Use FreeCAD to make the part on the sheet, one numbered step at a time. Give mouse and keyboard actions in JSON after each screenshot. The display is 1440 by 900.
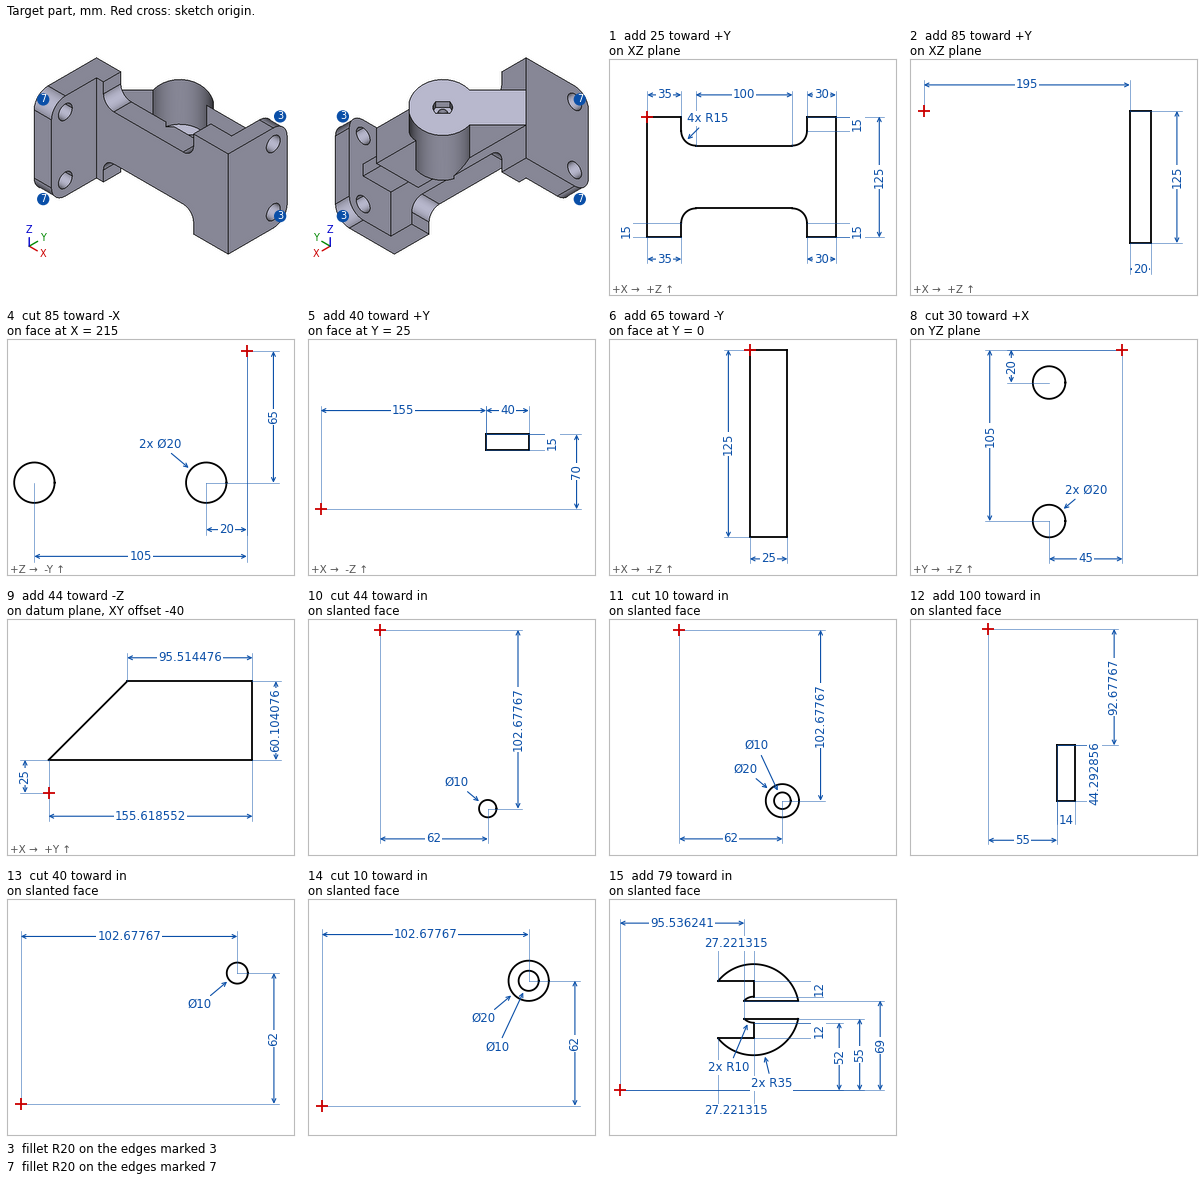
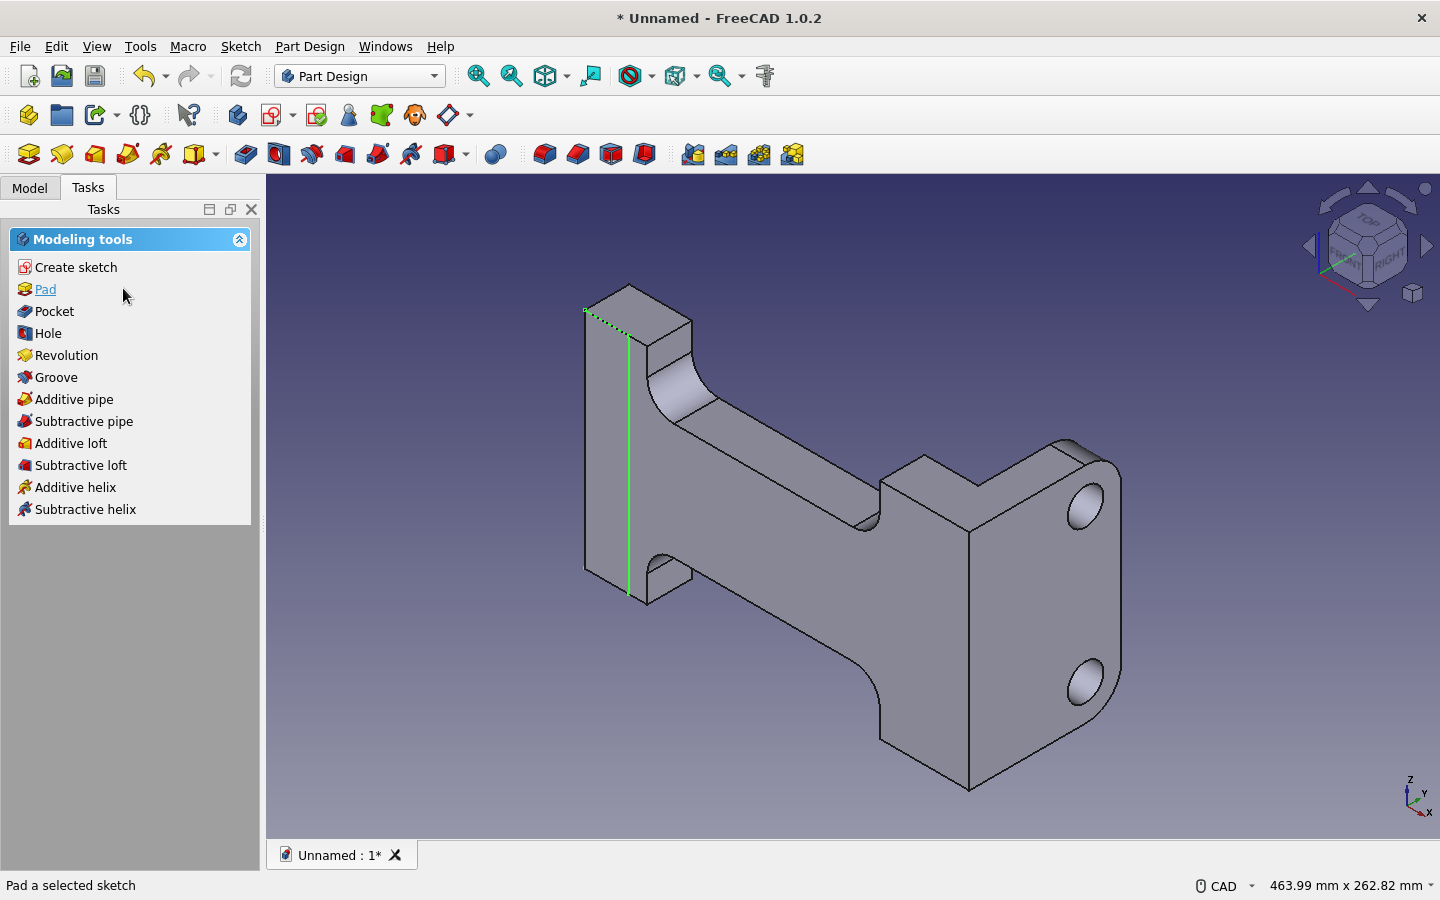
{"action": "left_click", "coordinate": [29, 154]}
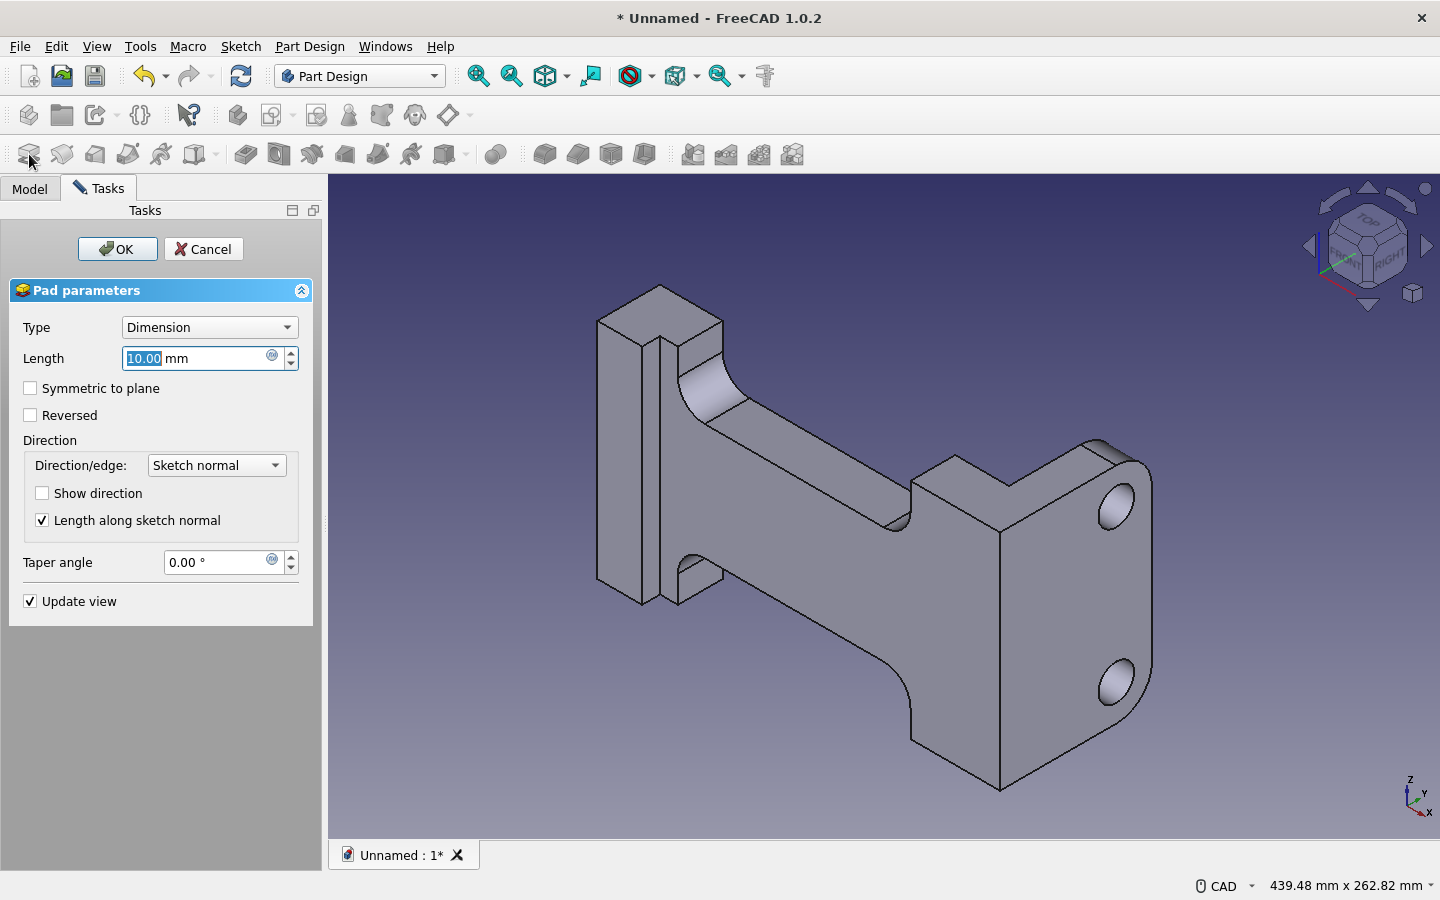
{"action": "type", "text": "65"}
{"action": "key", "text": "Tab"}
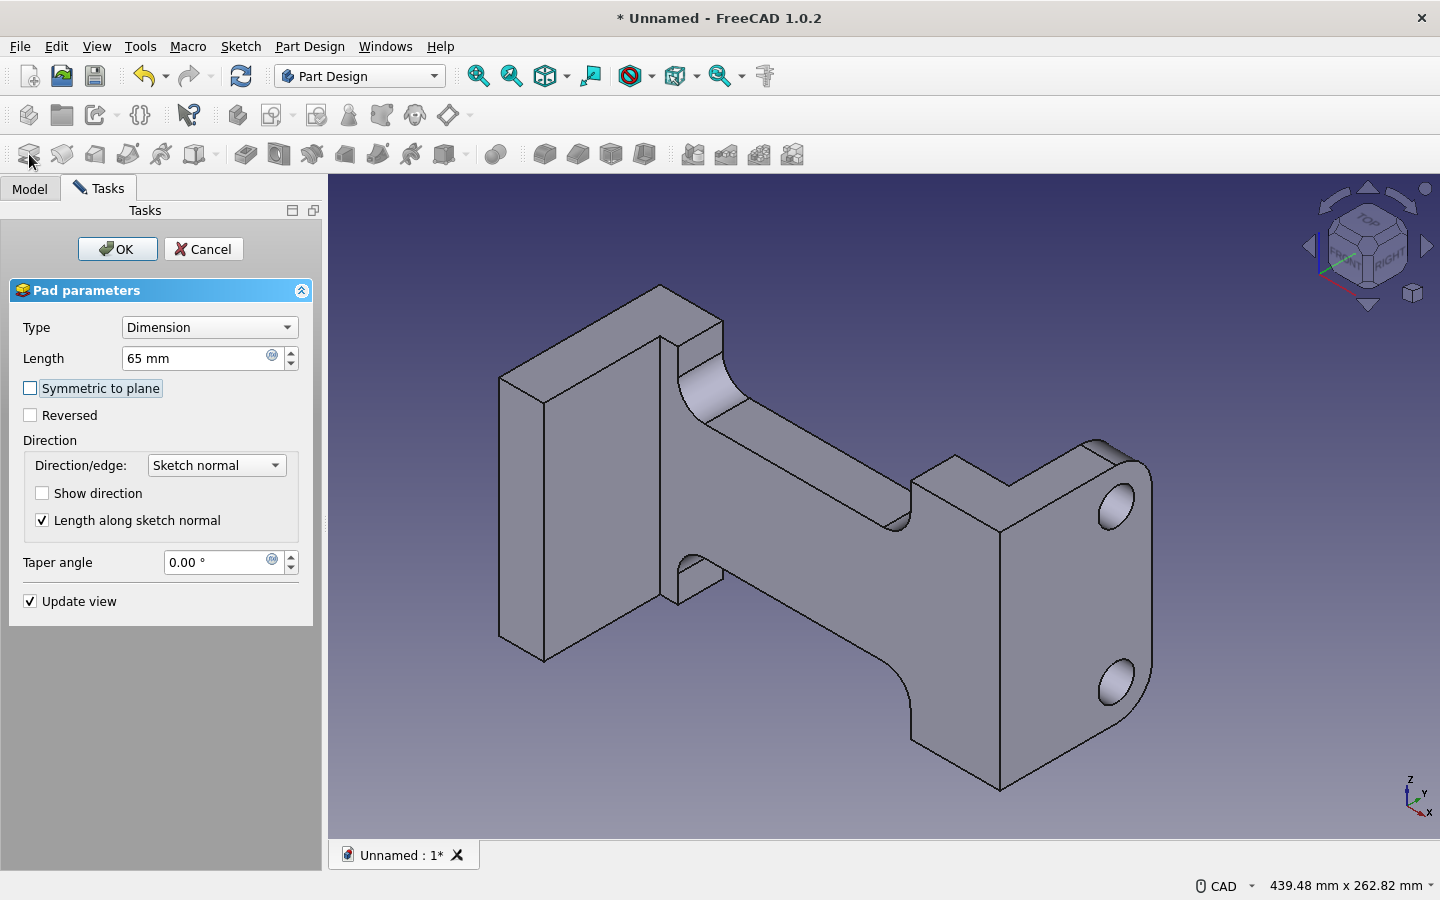
{"action": "left_click", "coordinate": [118, 249]}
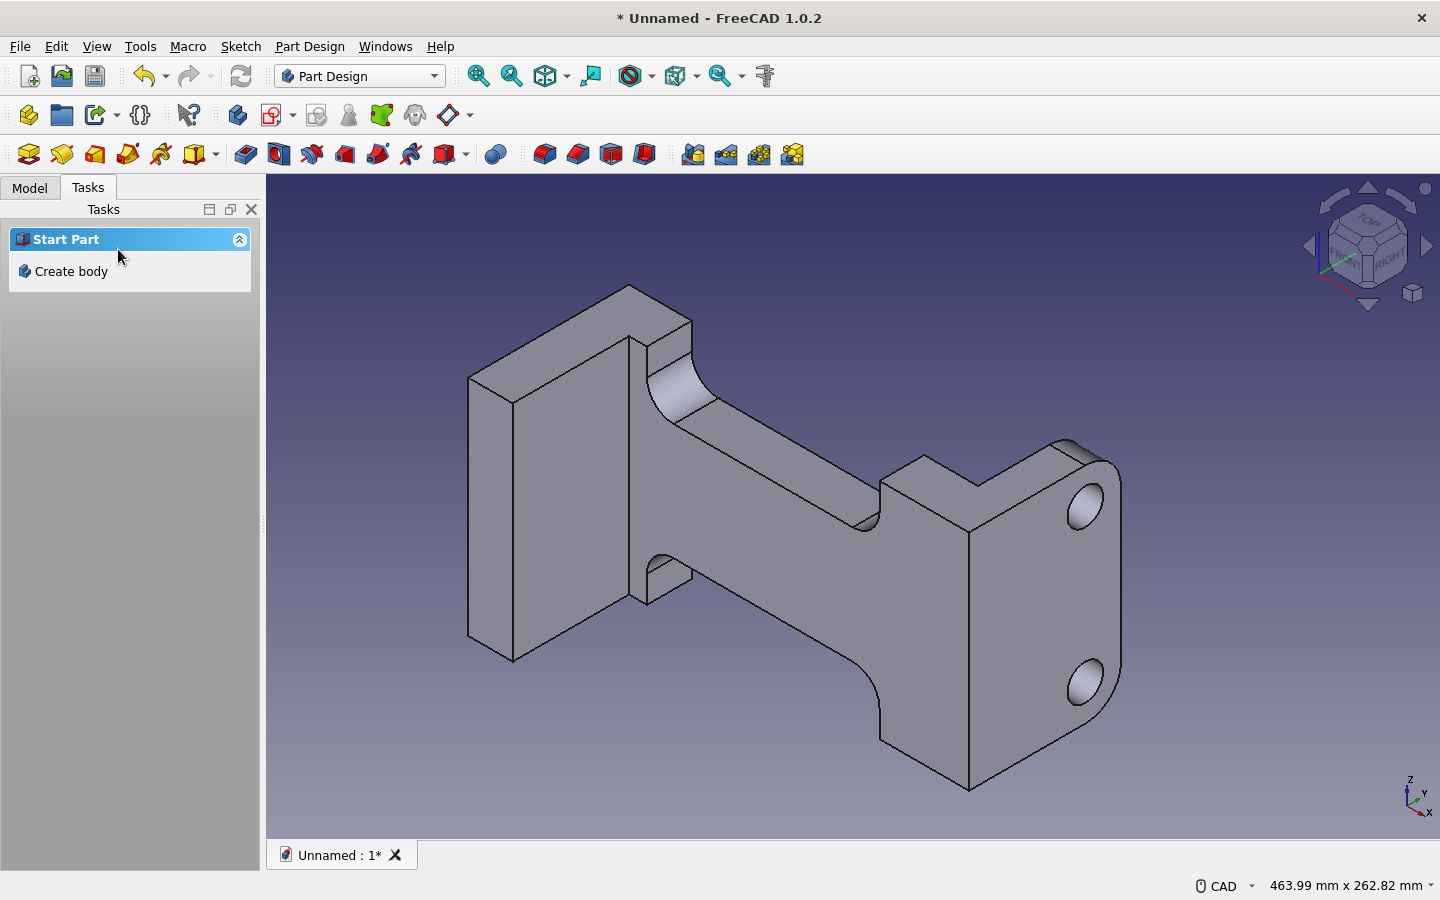
{"action": "key", "text": "v f"}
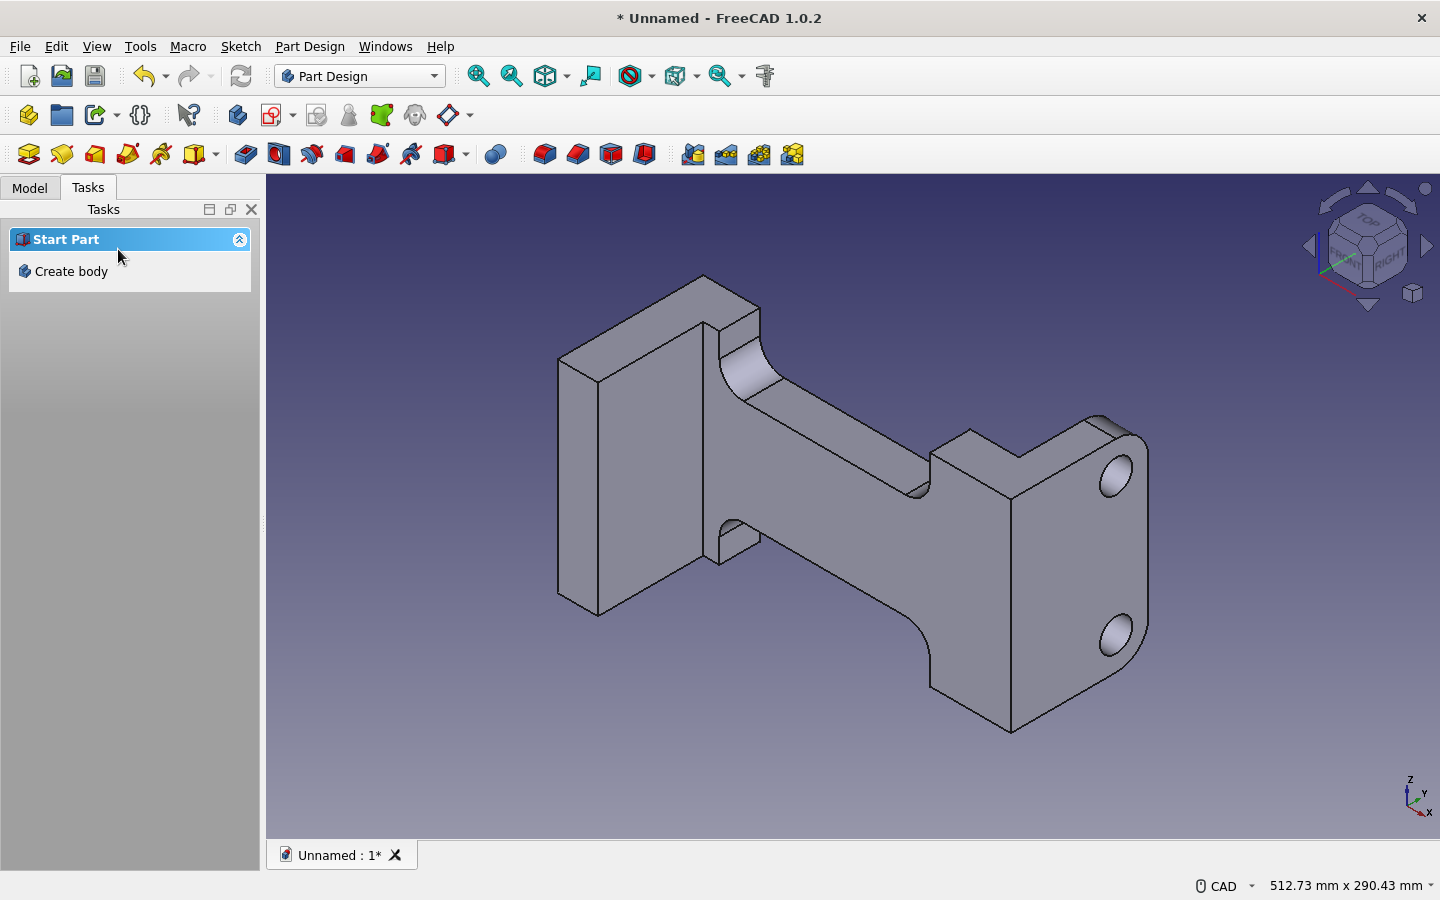
{"action": "left_click", "coordinate": [578, 370]}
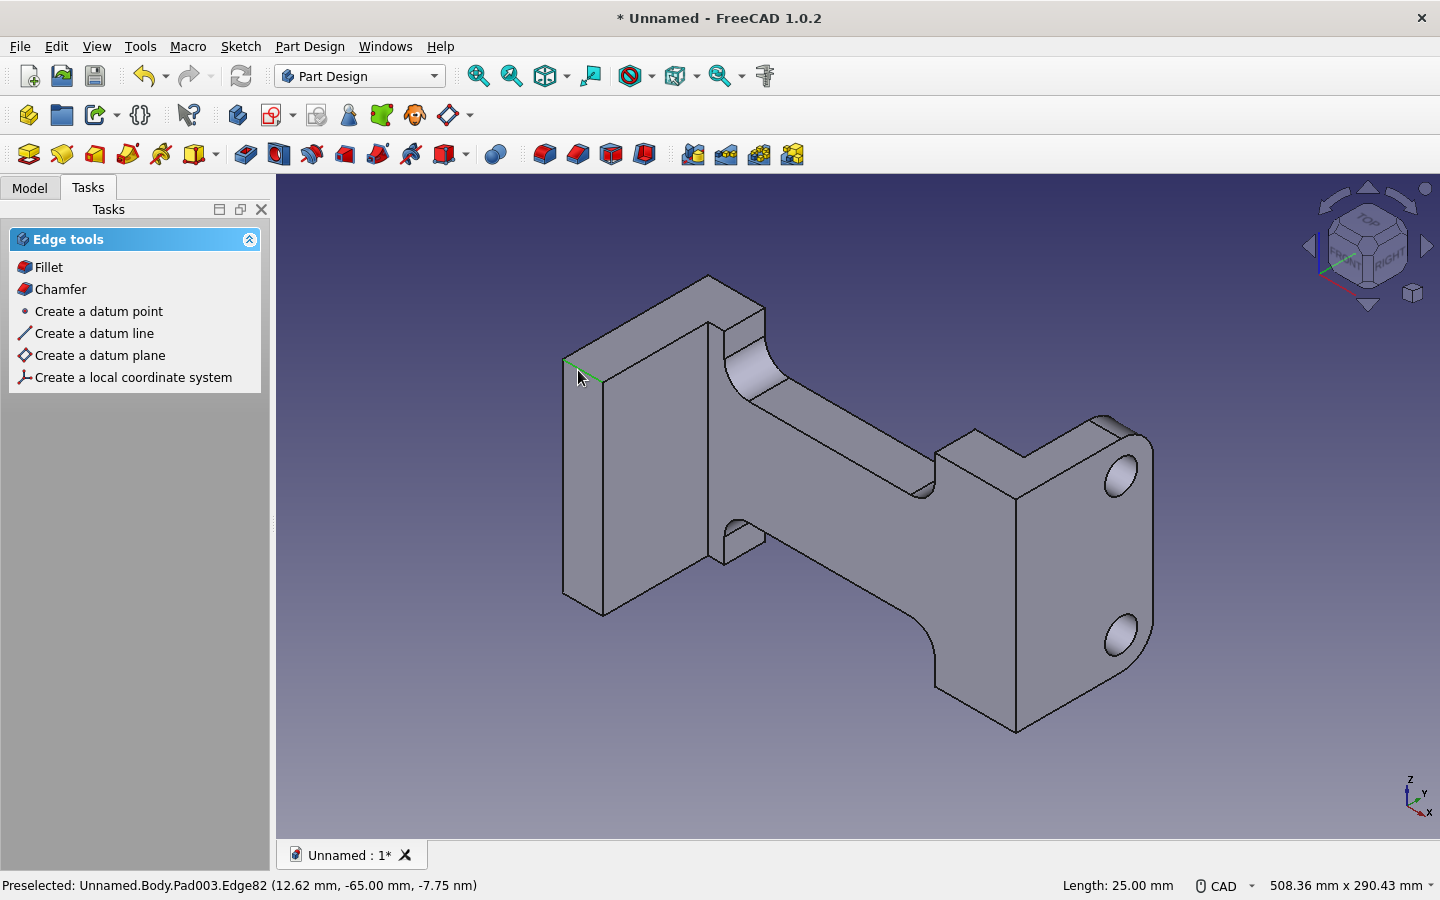
{"action": "key", "text": "2"}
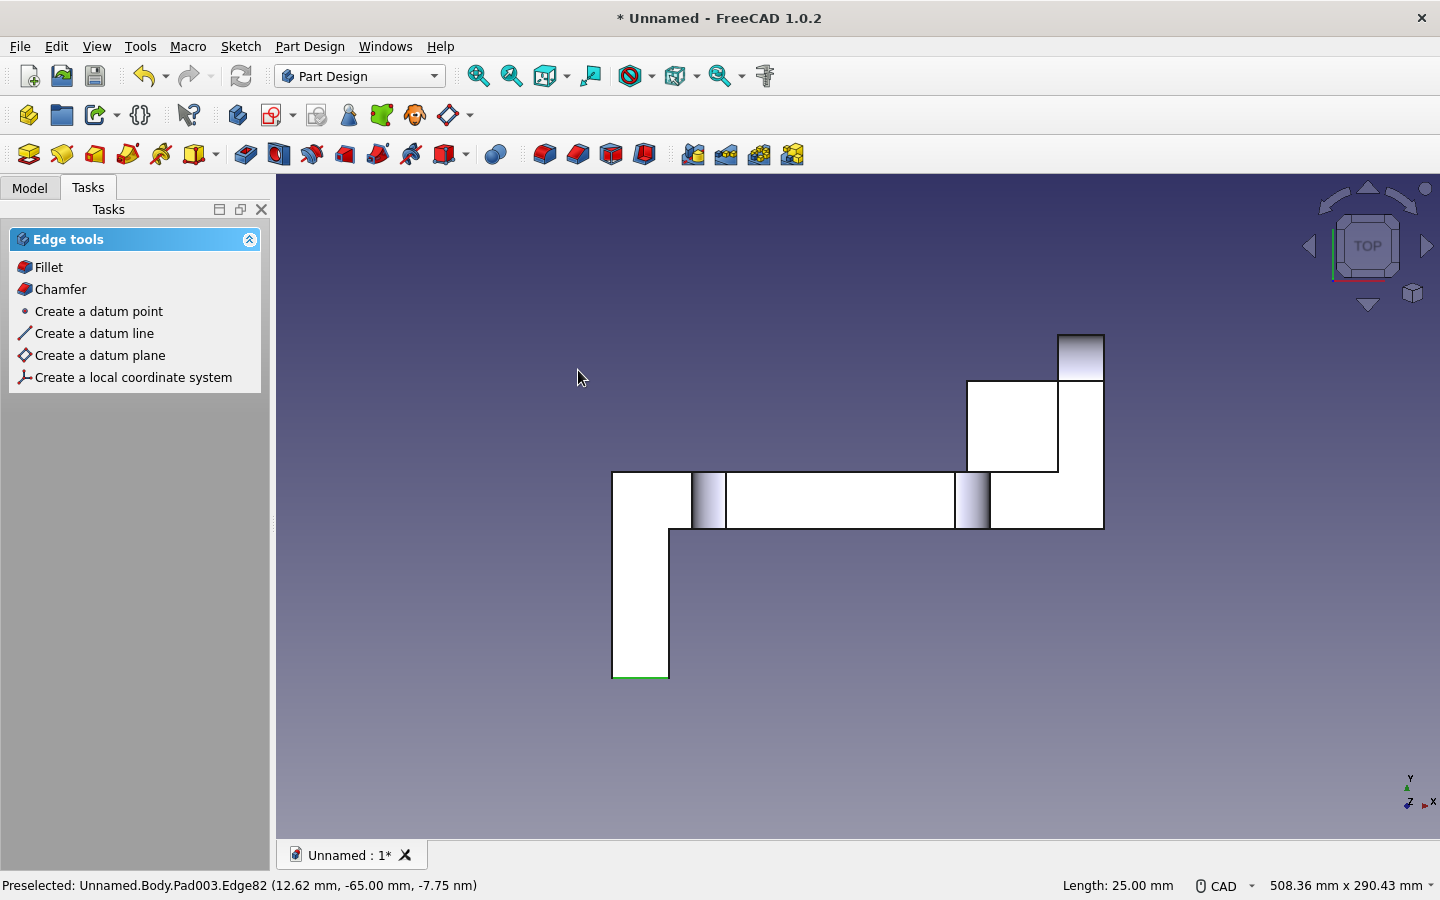
{"action": "key", "text": "0"}